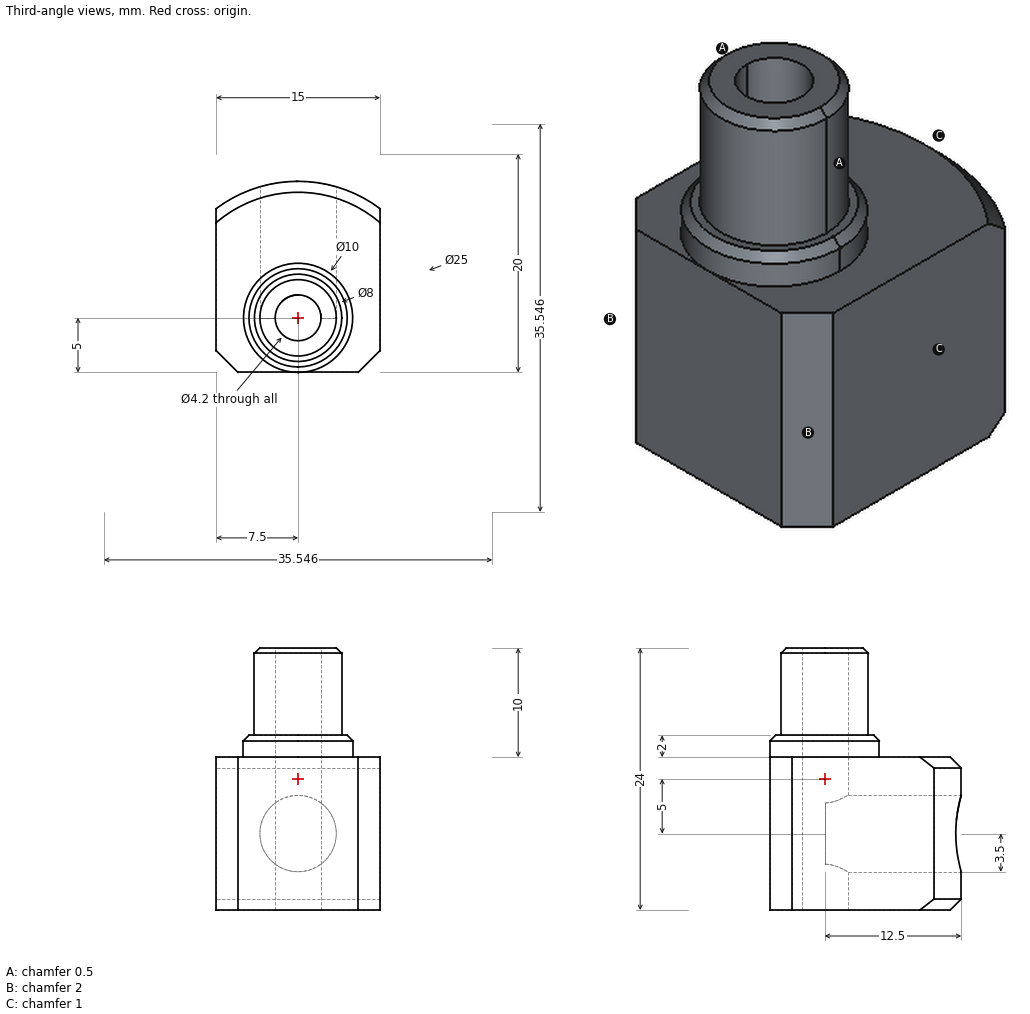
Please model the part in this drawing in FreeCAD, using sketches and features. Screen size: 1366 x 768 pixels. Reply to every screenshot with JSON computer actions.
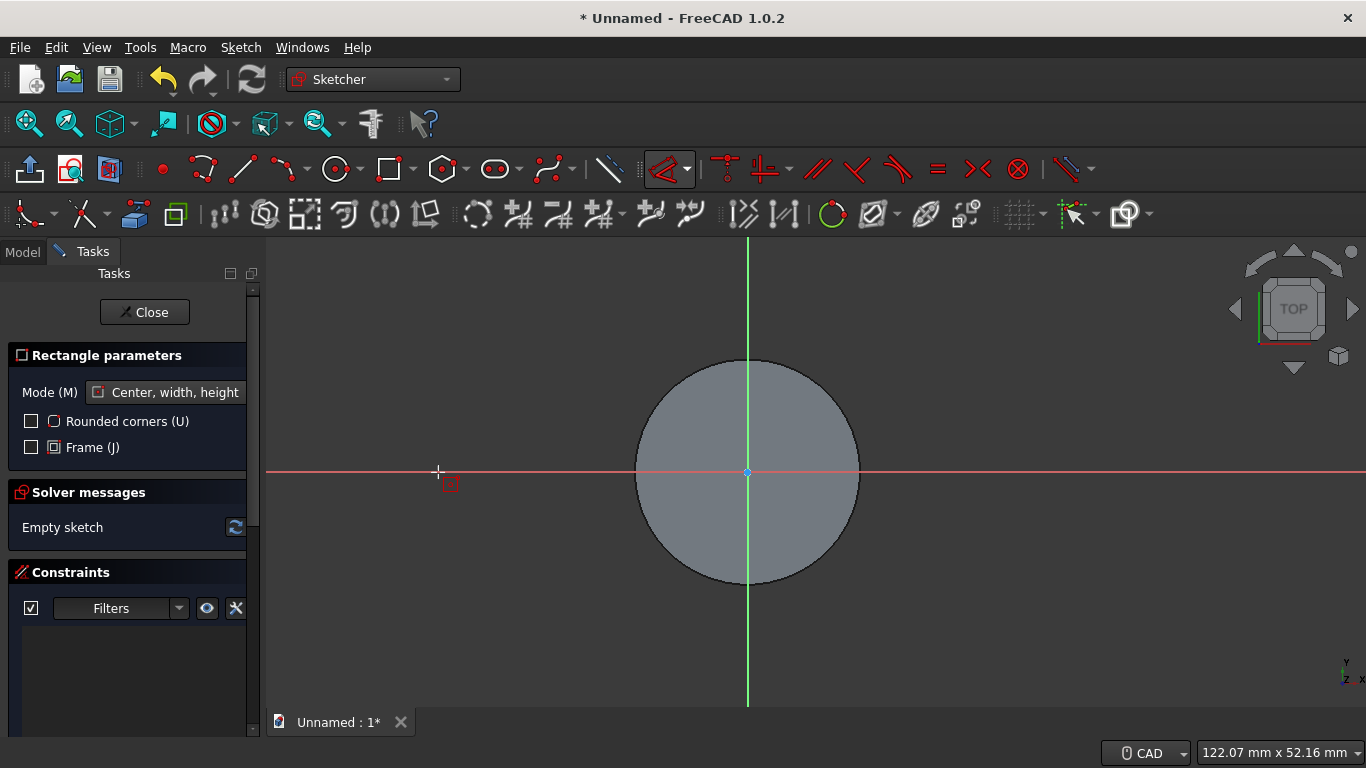
{"action": "left_click", "coordinate": [748, 472]}
{"action": "mouse_move", "coordinate": [908, 312]}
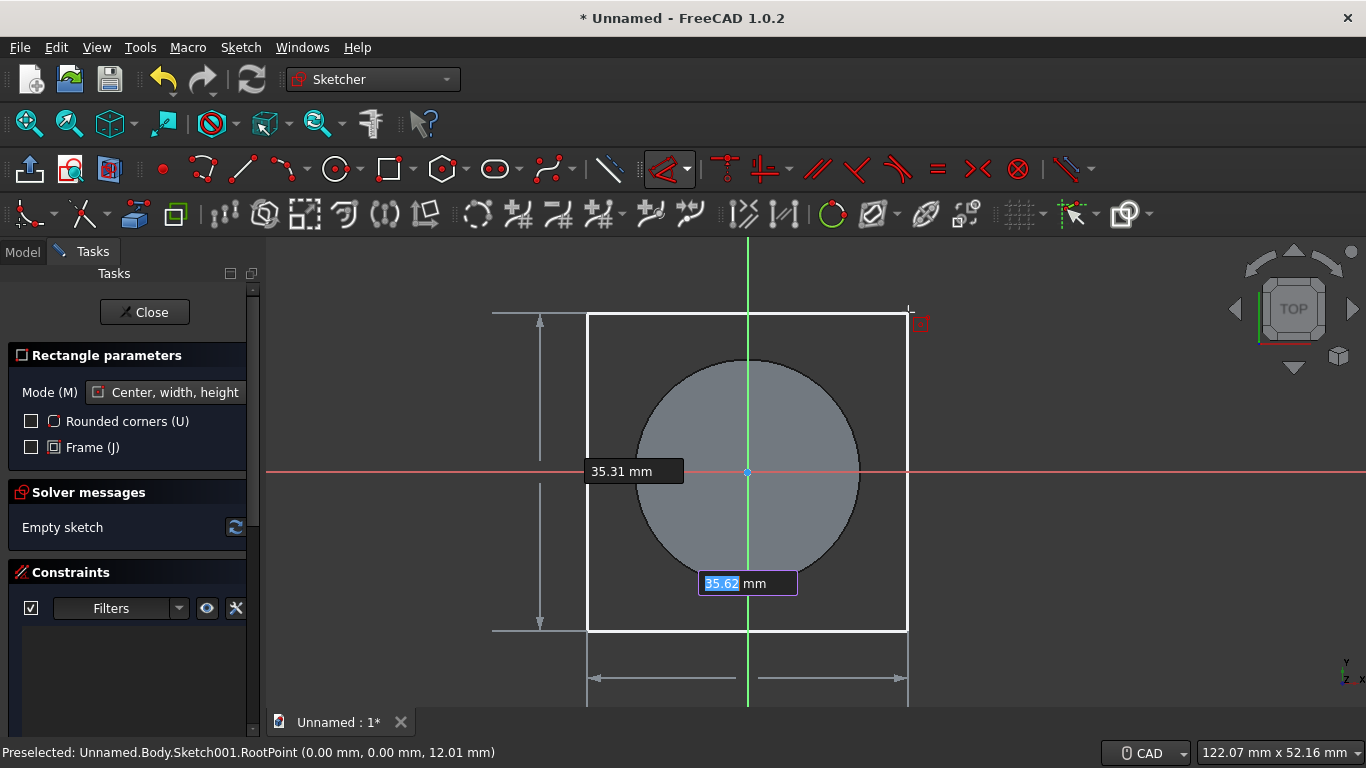
{"action": "type", "text": "35.546"}
{"action": "key", "text": "Tab"}
{"action": "type", "text": "35.546"}
{"action": "key", "text": "Return"}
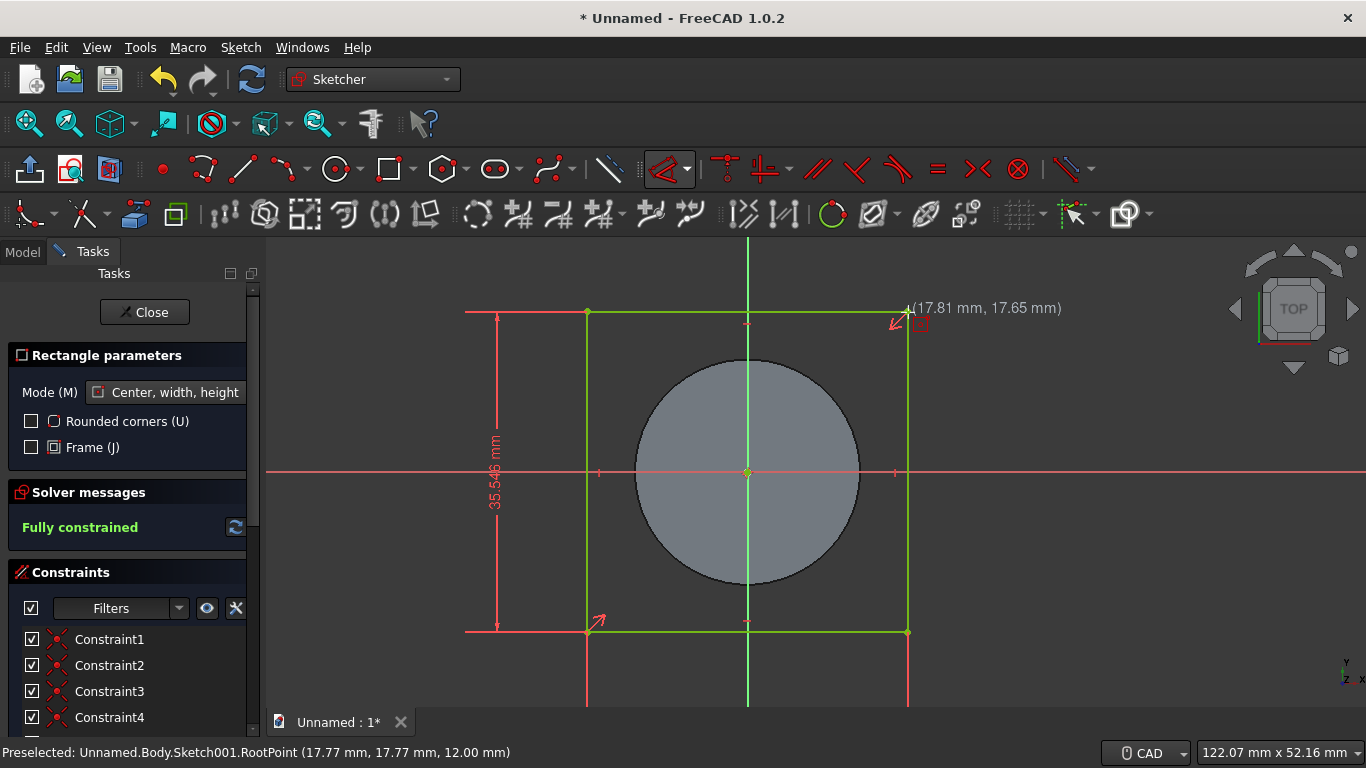
{"action": "key", "text": "g c"}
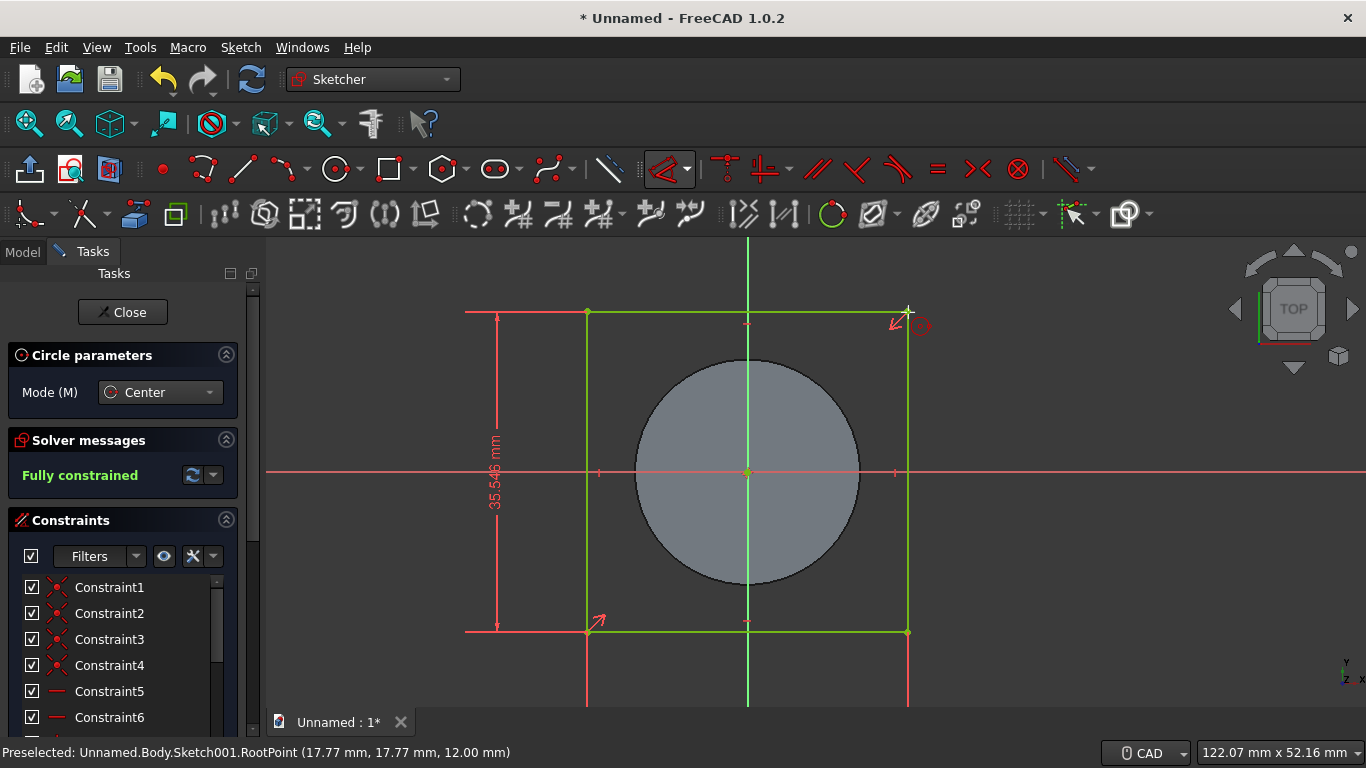
{"action": "left_click", "coordinate": [748, 472]}
{"action": "mouse_move", "coordinate": [773, 447]}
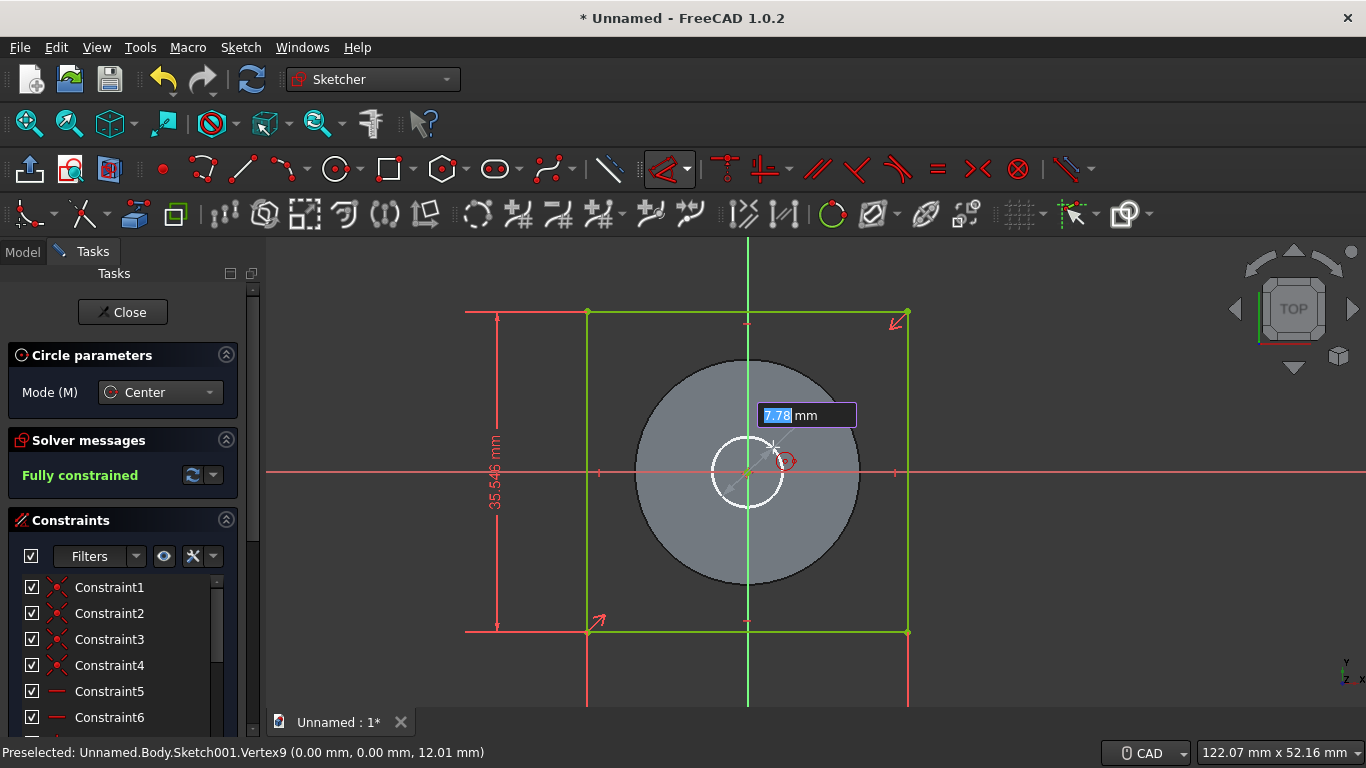
{"action": "type", "text": "8"}
{"action": "key", "text": "Return"}
{"action": "key", "text": "Escape"}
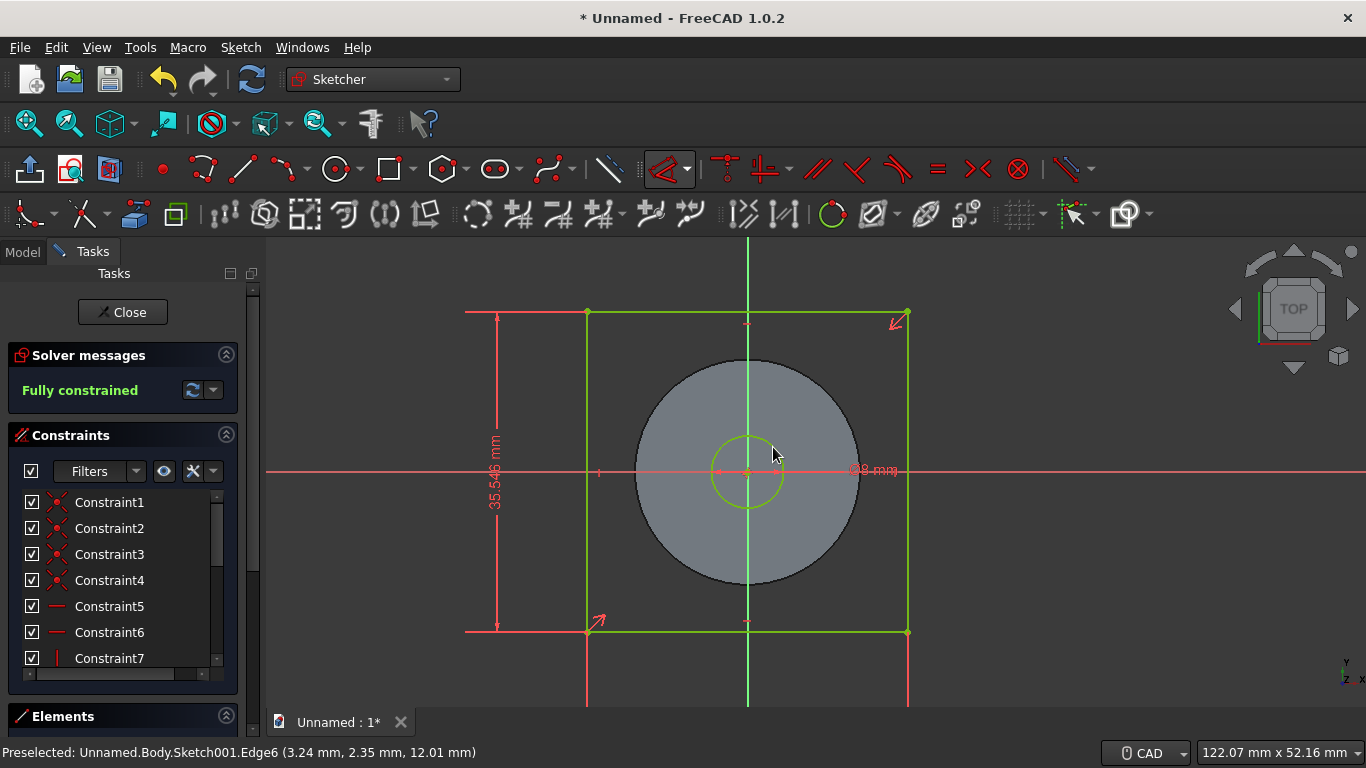
{"action": "left_click", "coordinate": [123, 312]}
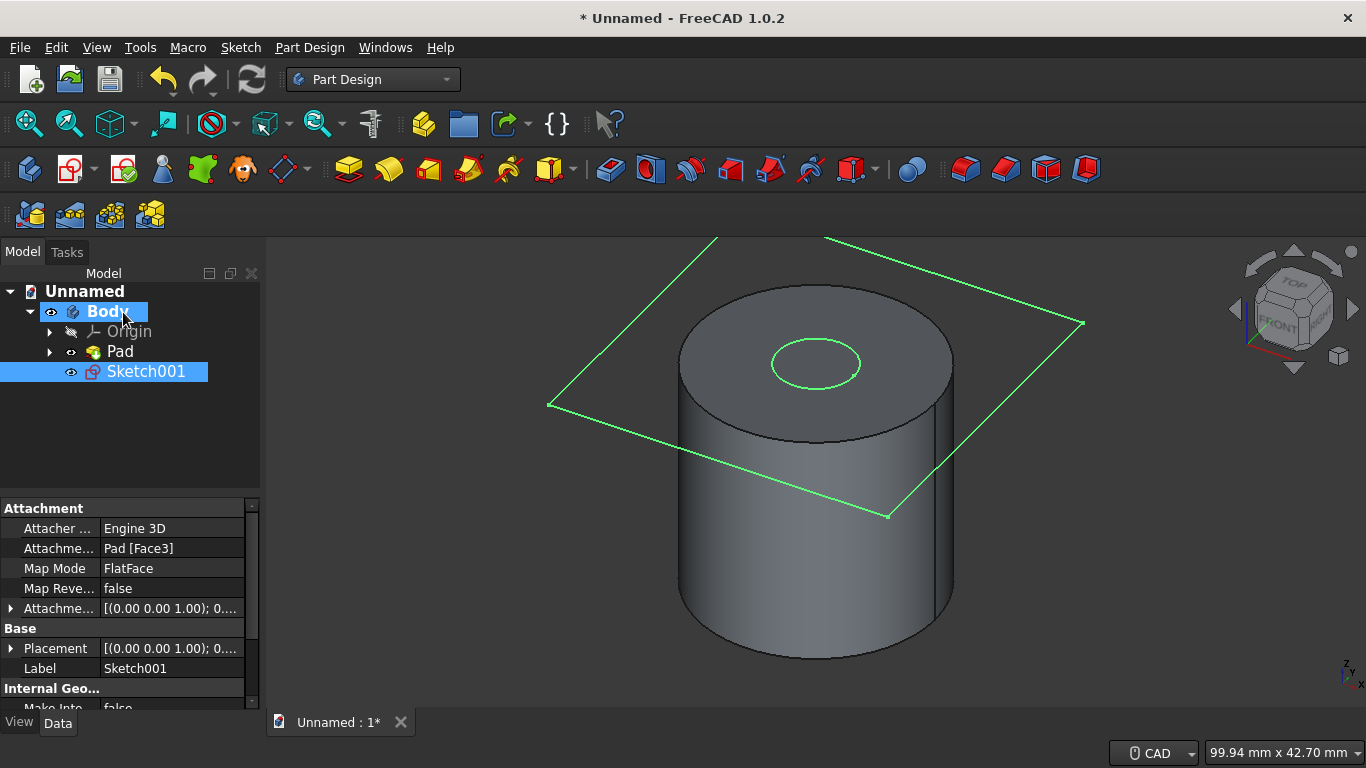
{"action": "left_click", "coordinate": [612, 170]}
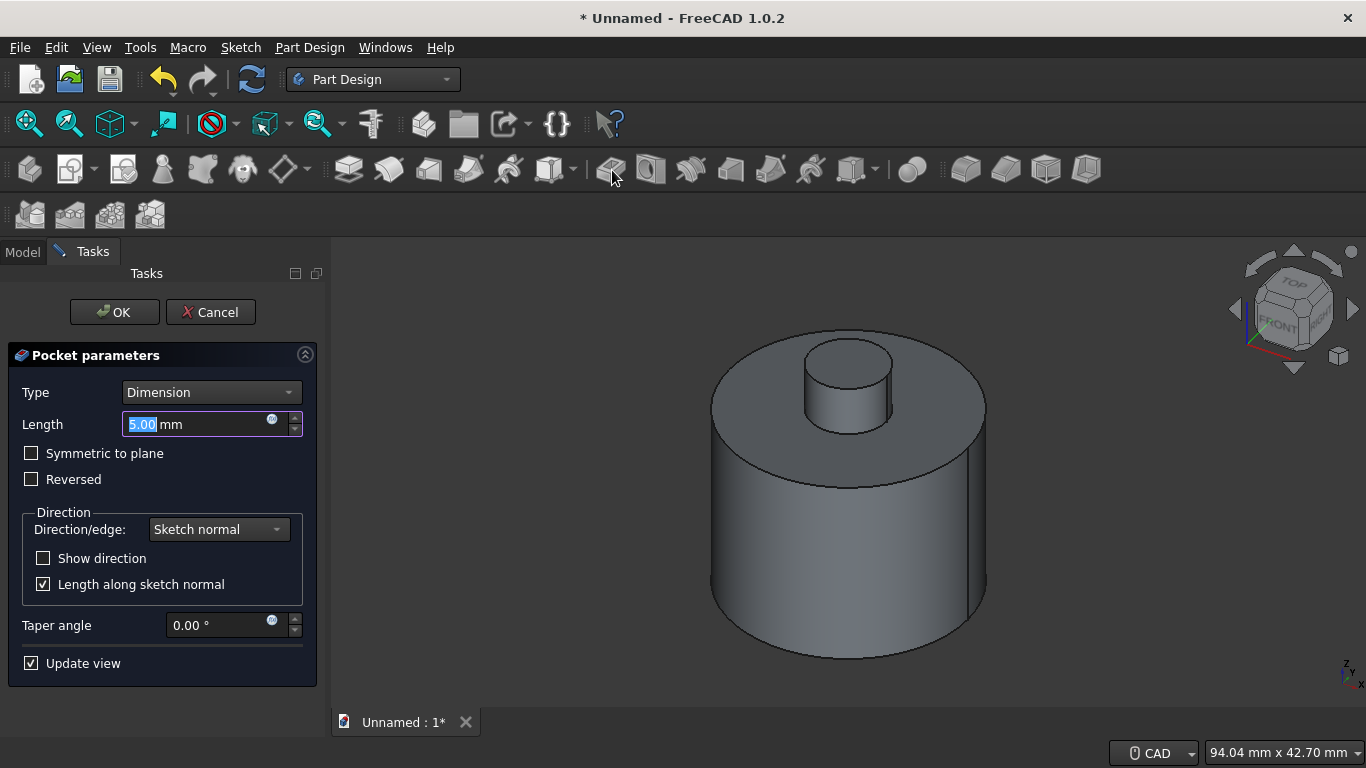
{"action": "type", "text": "10"}
{"action": "key", "text": "Tab"}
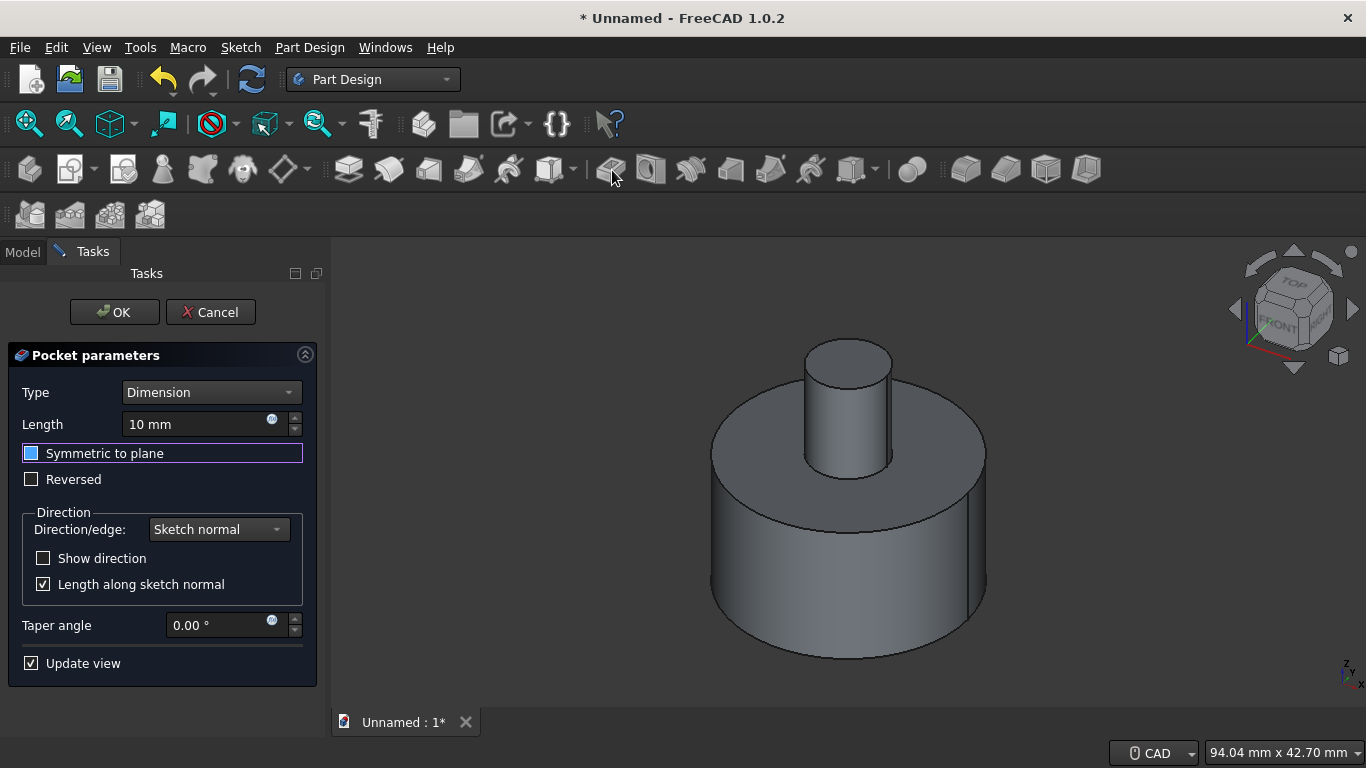
{"action": "left_click", "coordinate": [115, 312]}